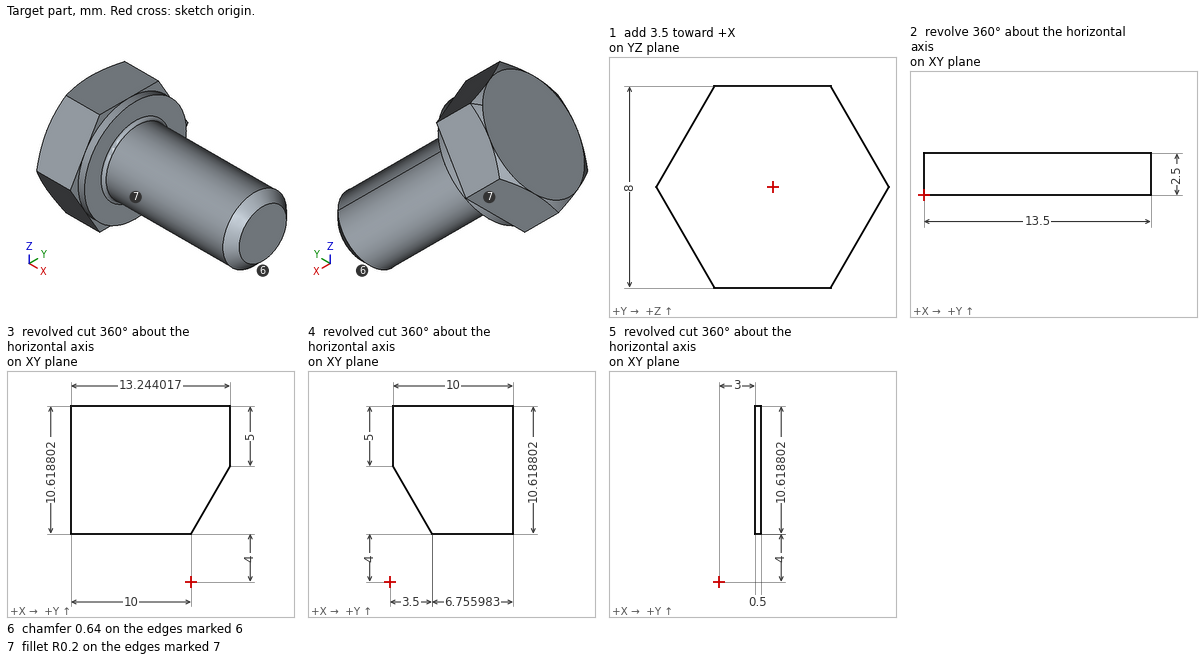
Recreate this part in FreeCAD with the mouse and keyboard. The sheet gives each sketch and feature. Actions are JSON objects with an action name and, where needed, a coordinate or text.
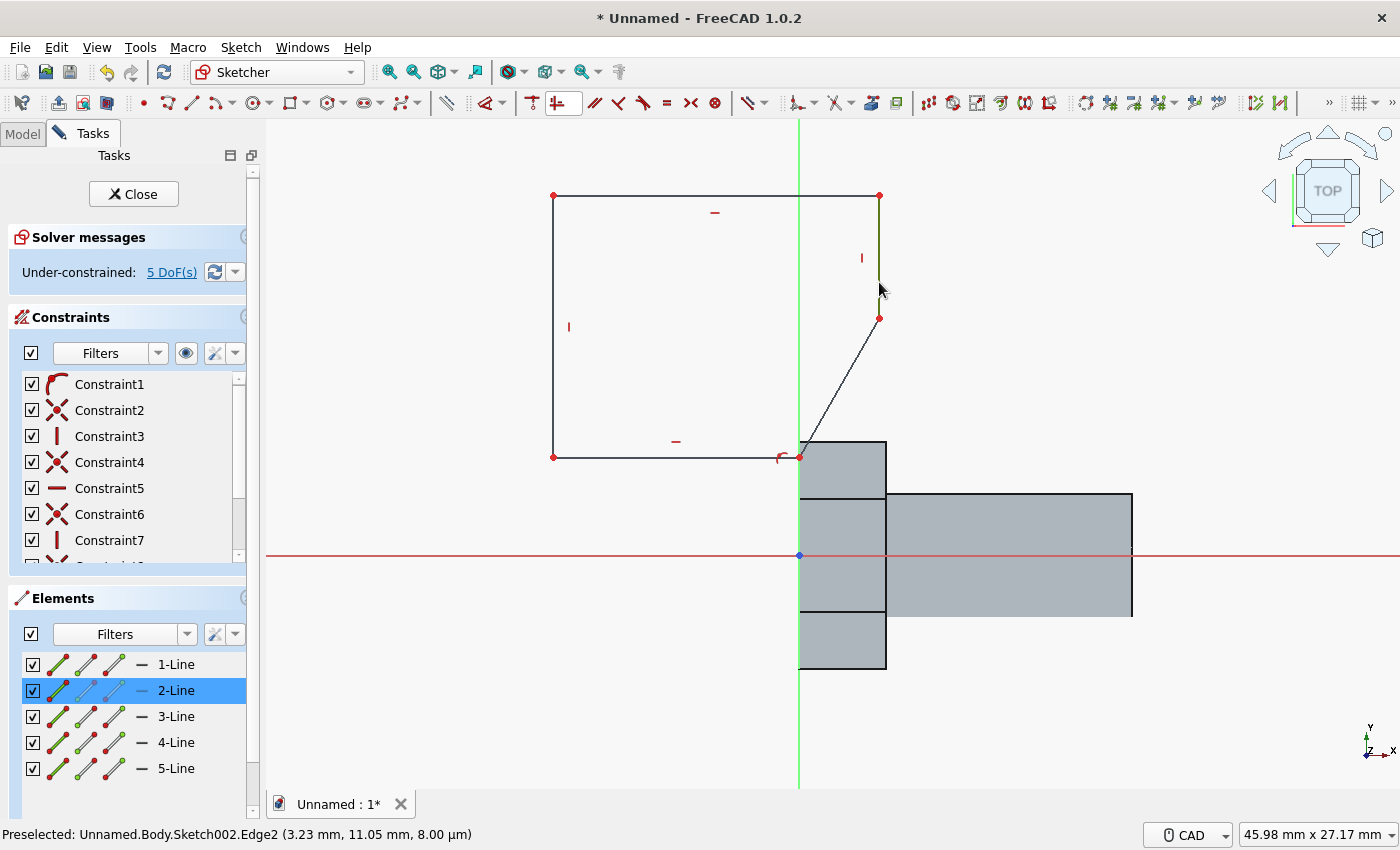
{"action": "left_click", "coordinate": [504, 104]}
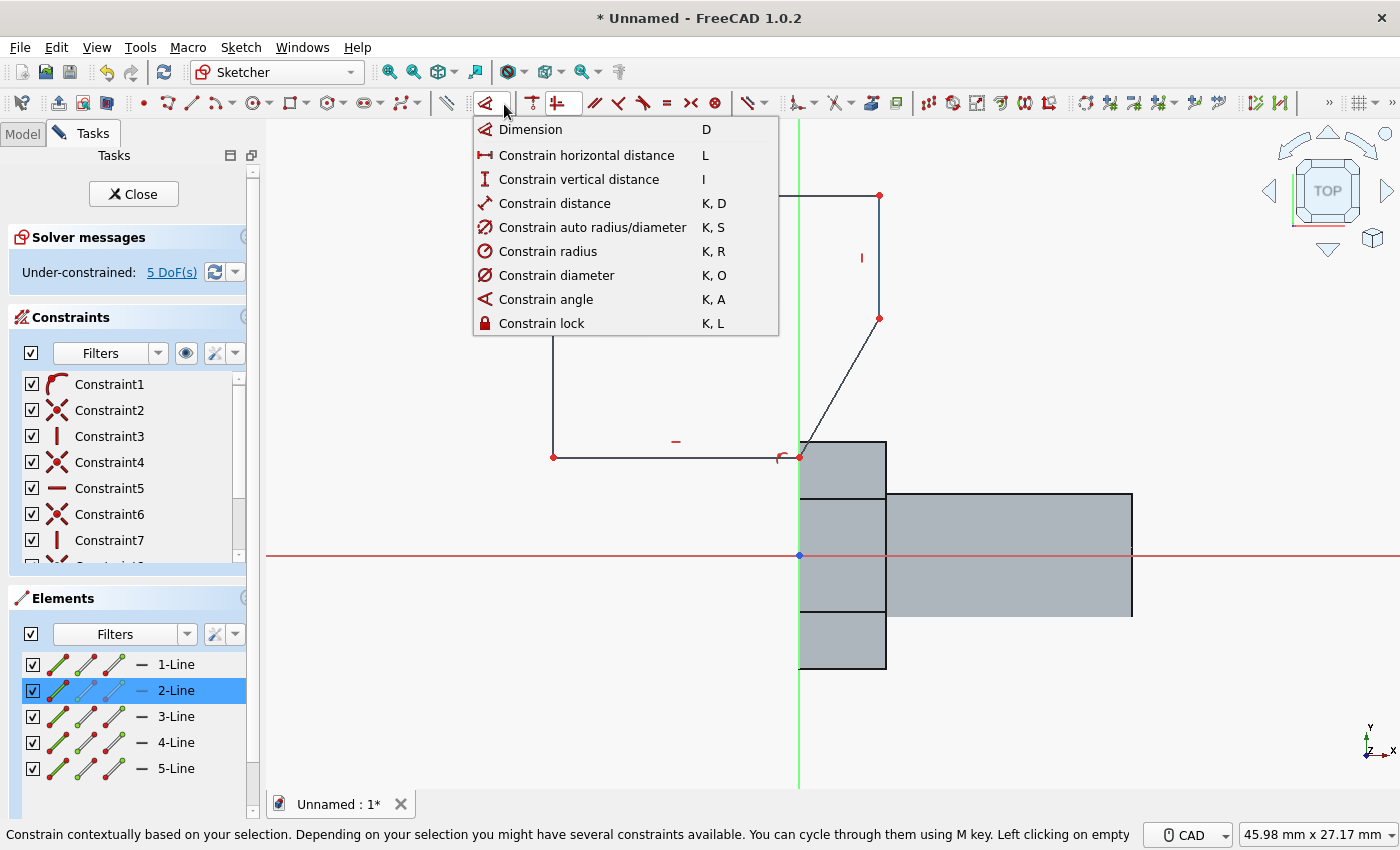
{"action": "left_click", "coordinate": [626, 179]}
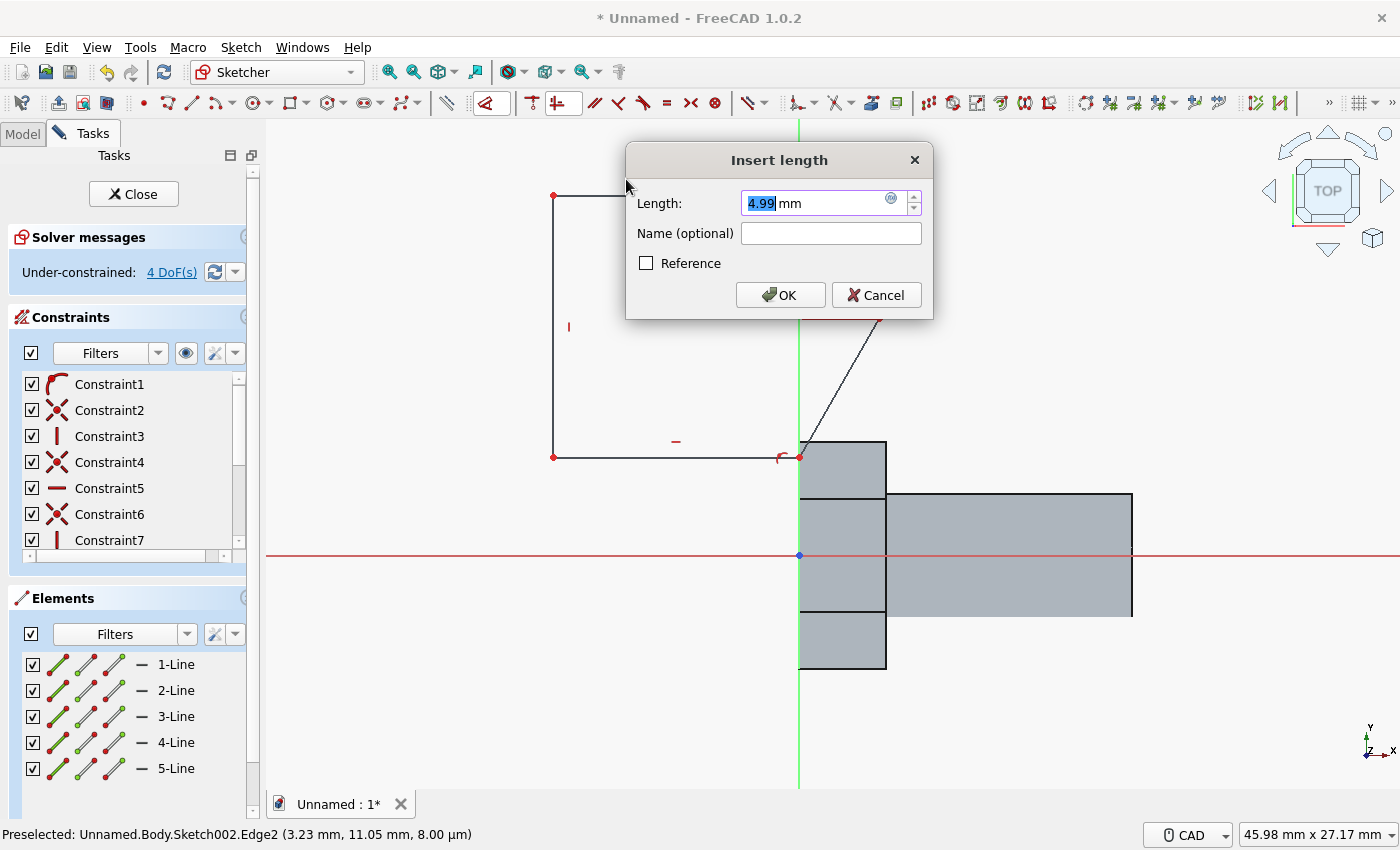
{"action": "type", "text": "5"}
{"action": "key", "text": "Return"}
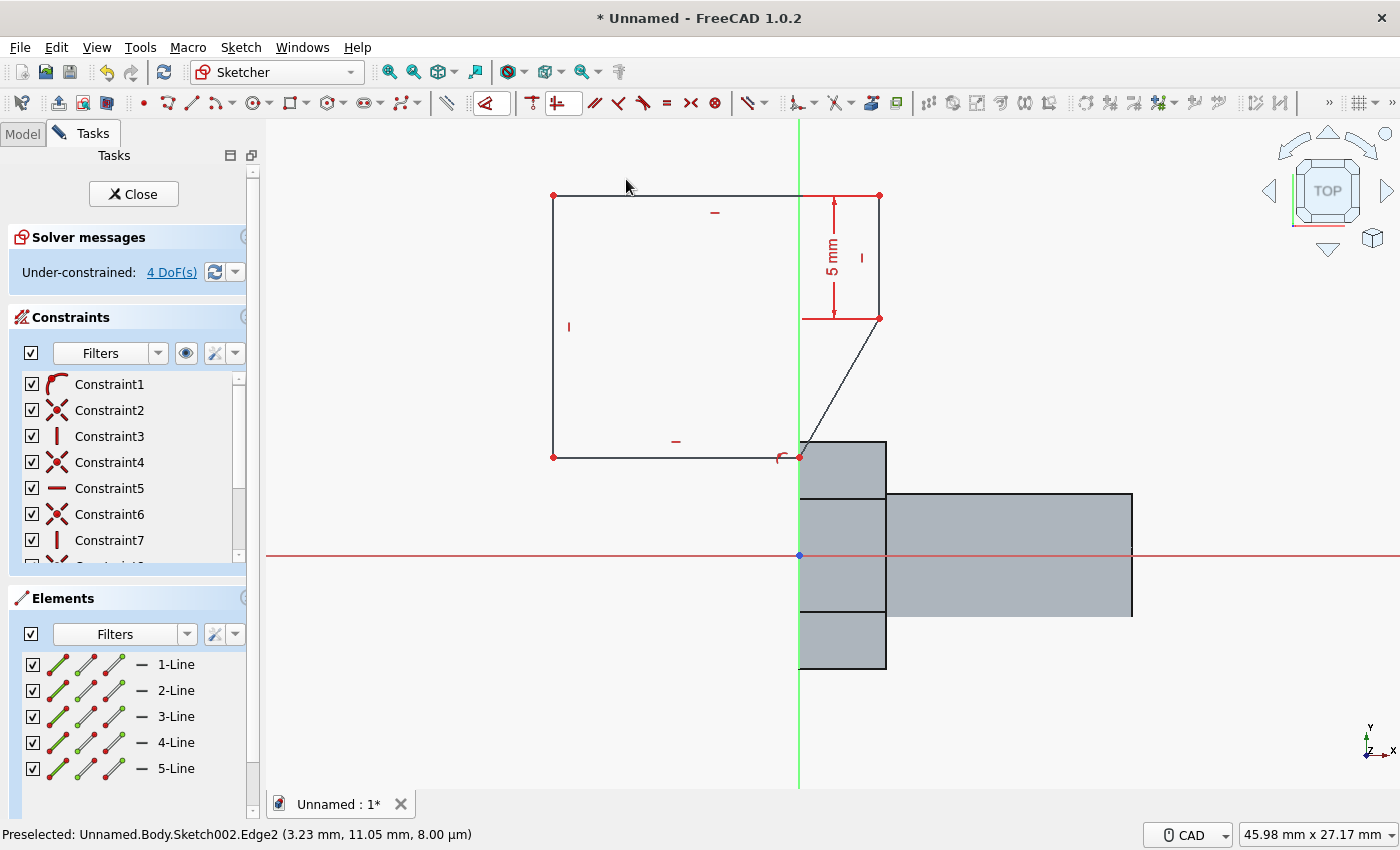
{"action": "left_click", "coordinate": [627, 458]}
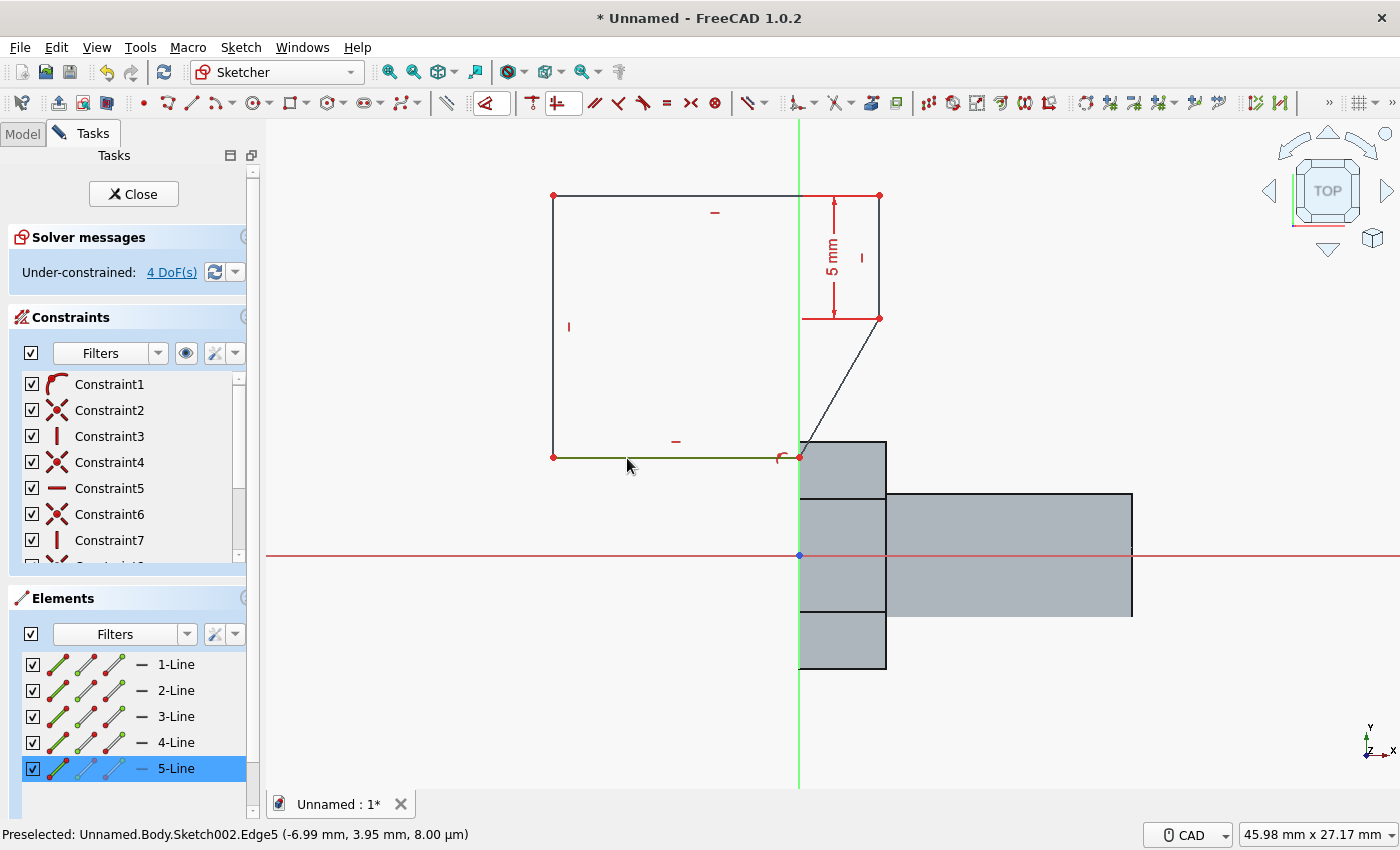
{"action": "left_click", "coordinate": [504, 104]}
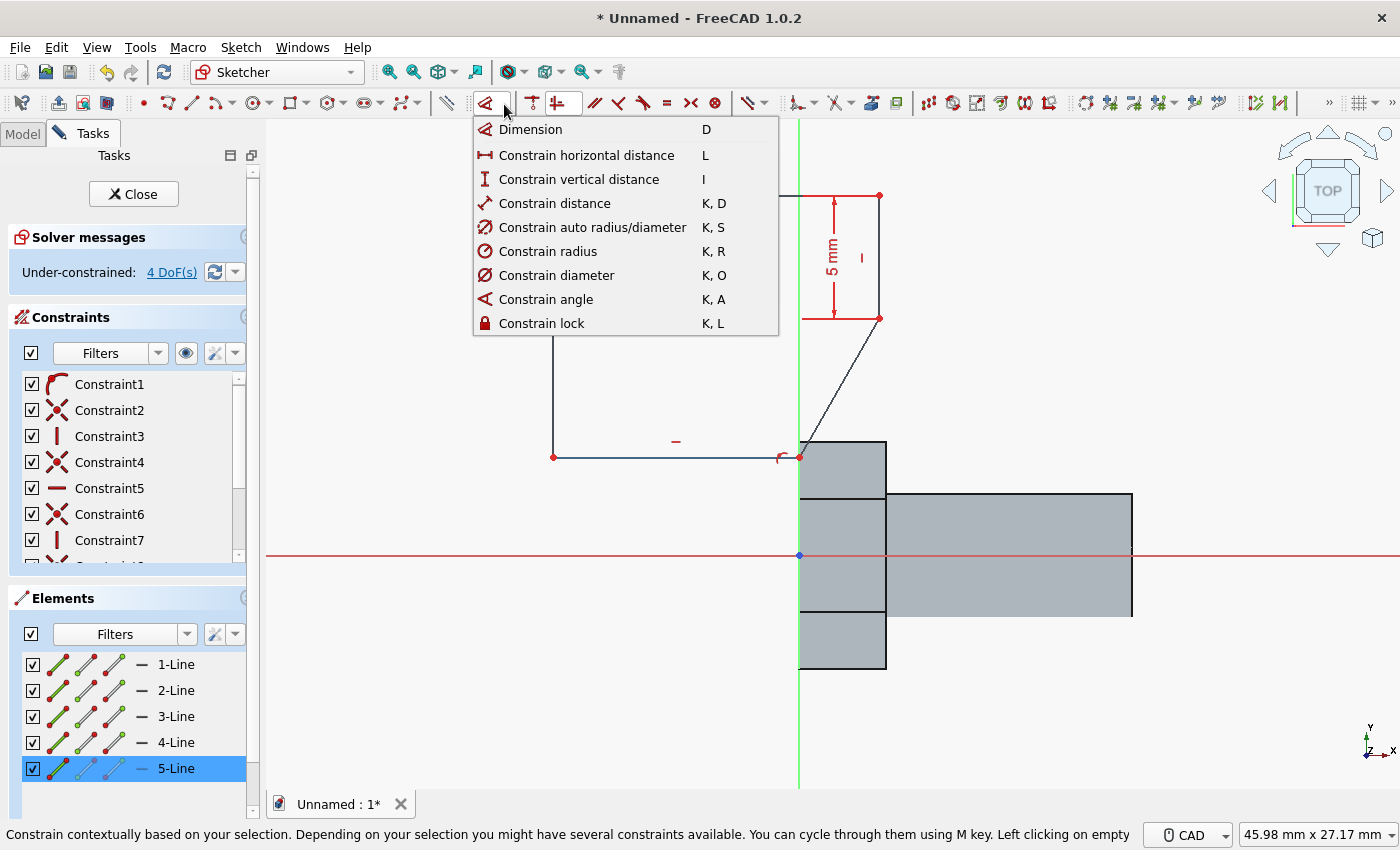
{"action": "left_click", "coordinate": [626, 155]}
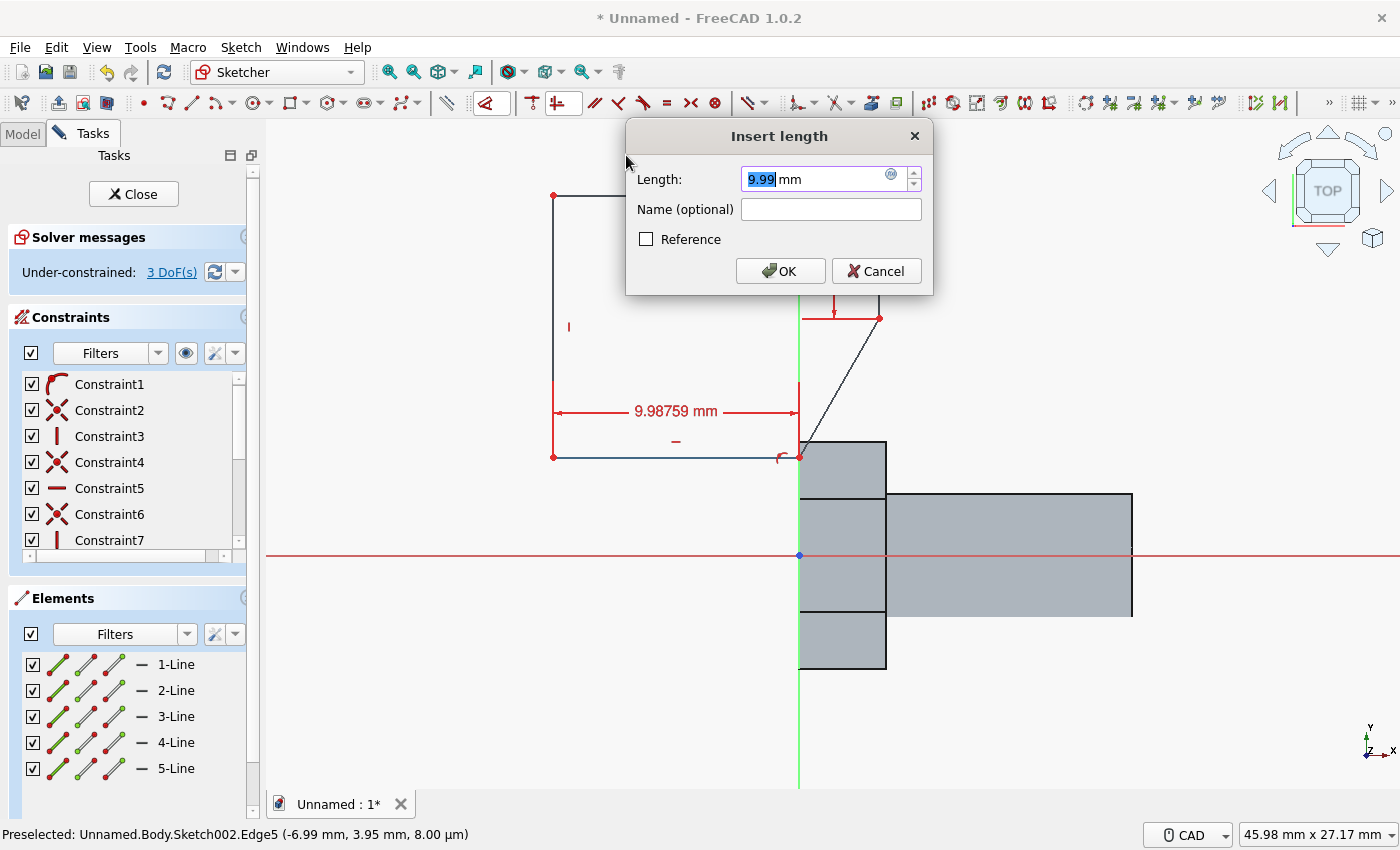
{"action": "type", "text": "10"}
{"action": "key", "text": "Return"}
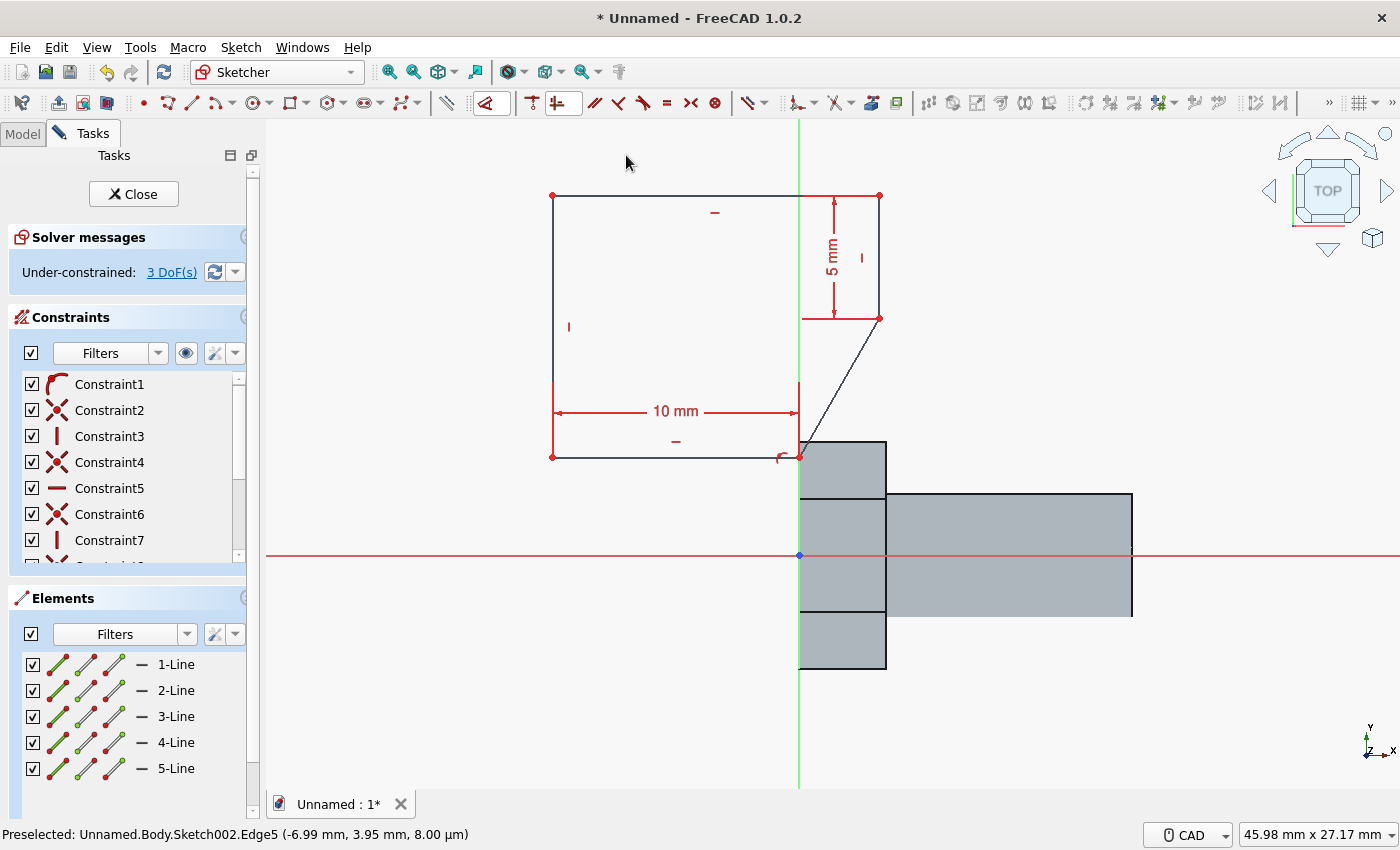
{"action": "left_click", "coordinate": [799, 458]}